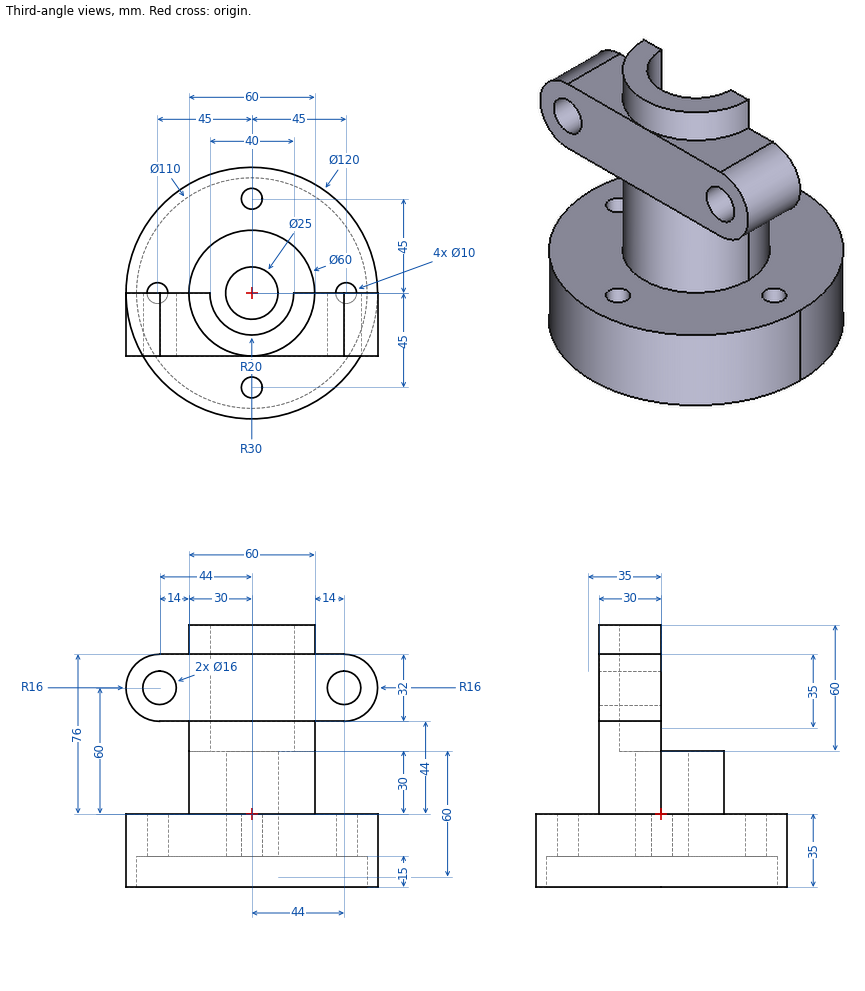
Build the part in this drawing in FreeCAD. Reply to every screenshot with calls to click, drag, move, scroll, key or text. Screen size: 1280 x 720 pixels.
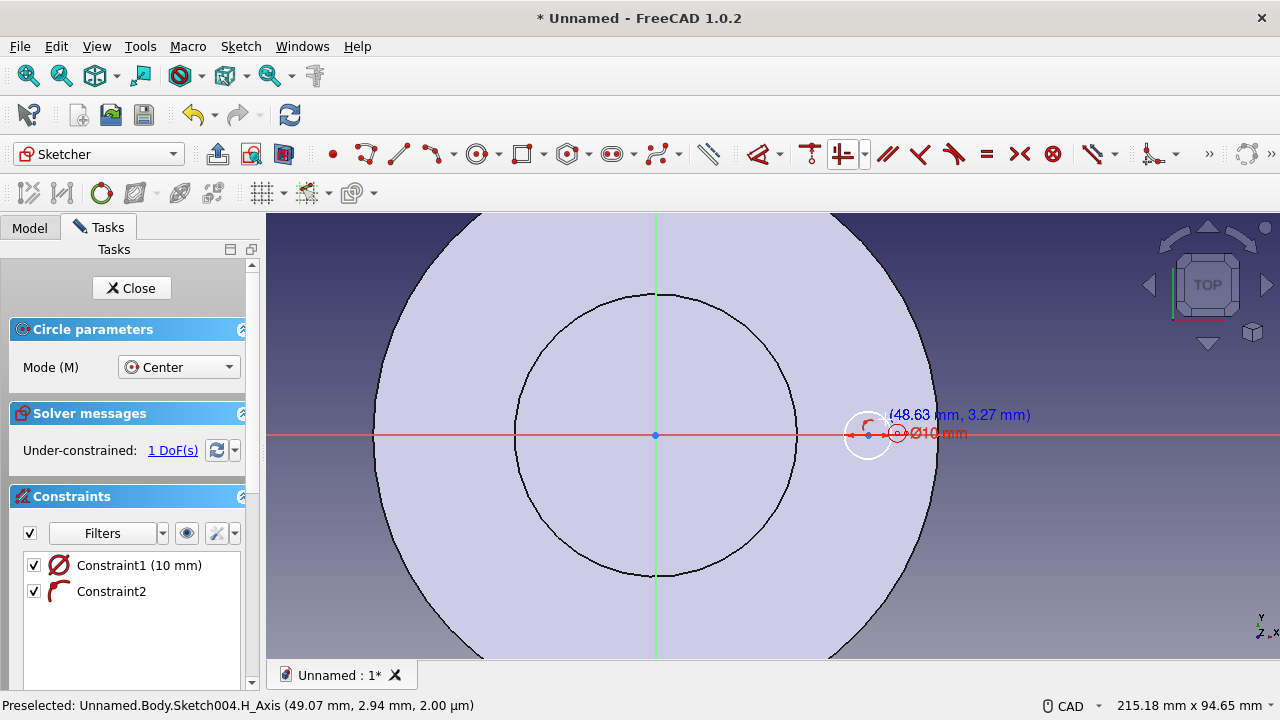
scroll(764, 437, down, 3)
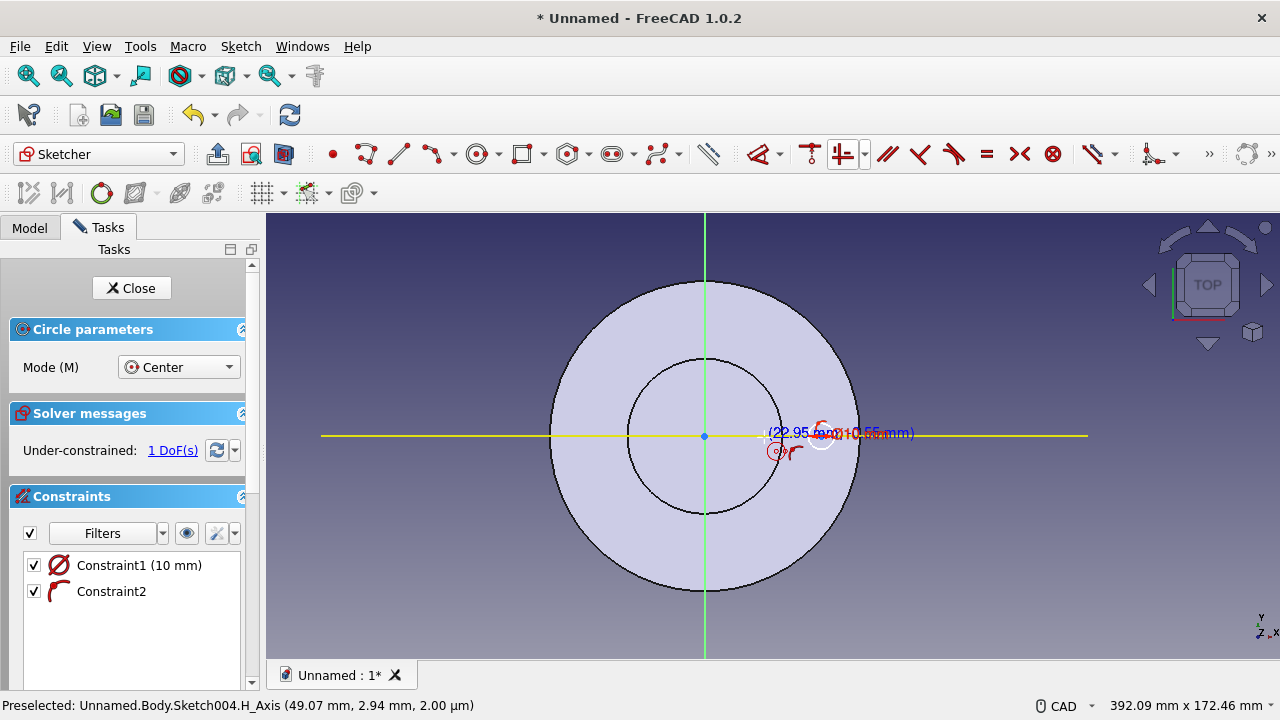
scroll(705, 320, up, 3)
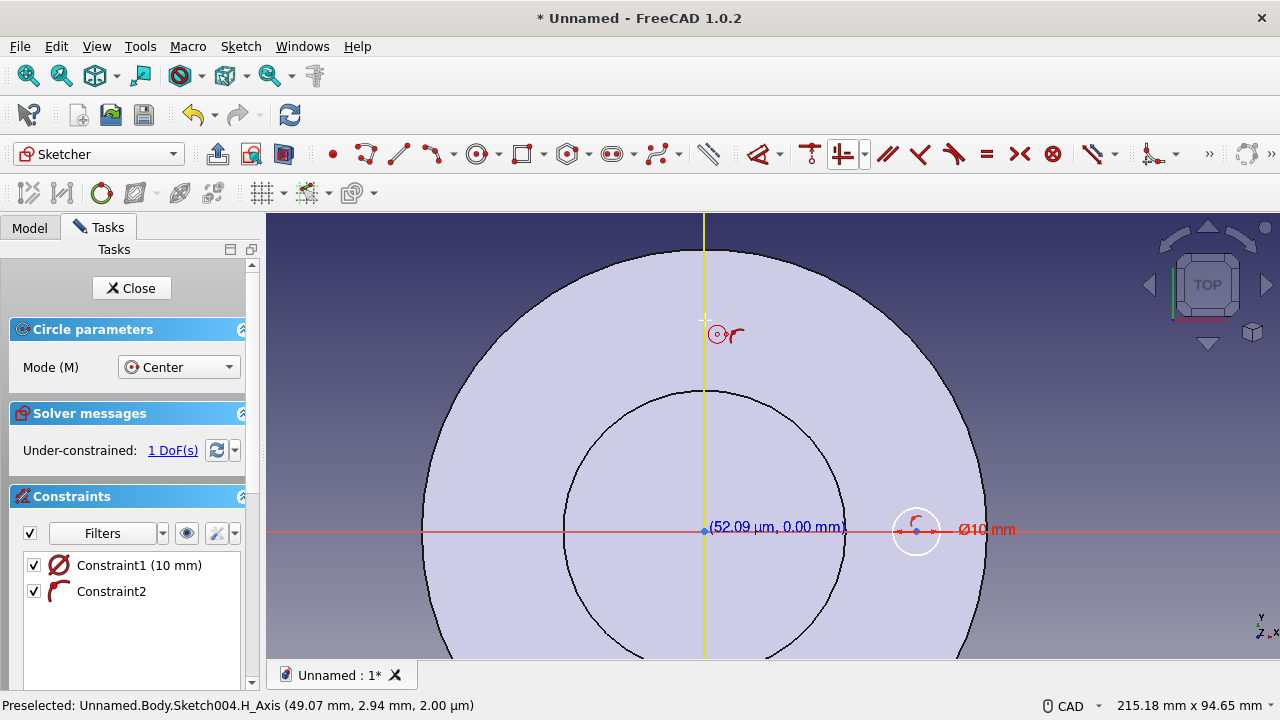
click(704, 320)
move(721, 303)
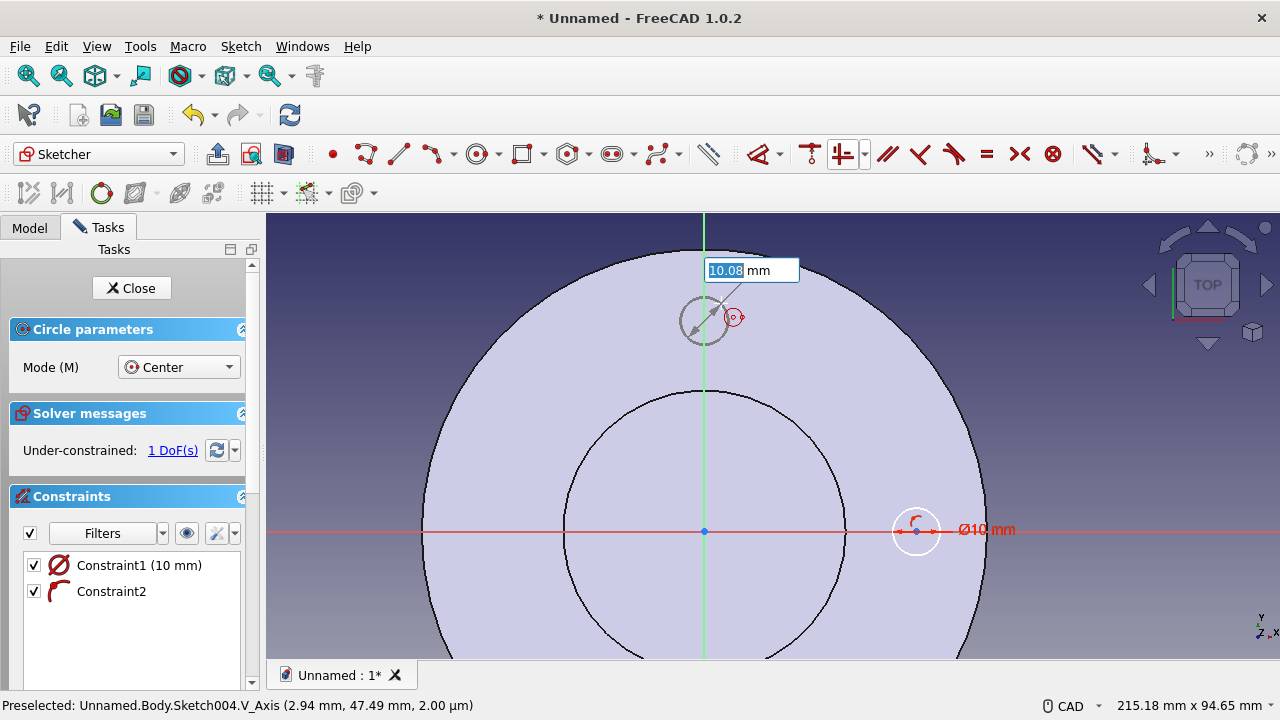
text(10)
key(Return)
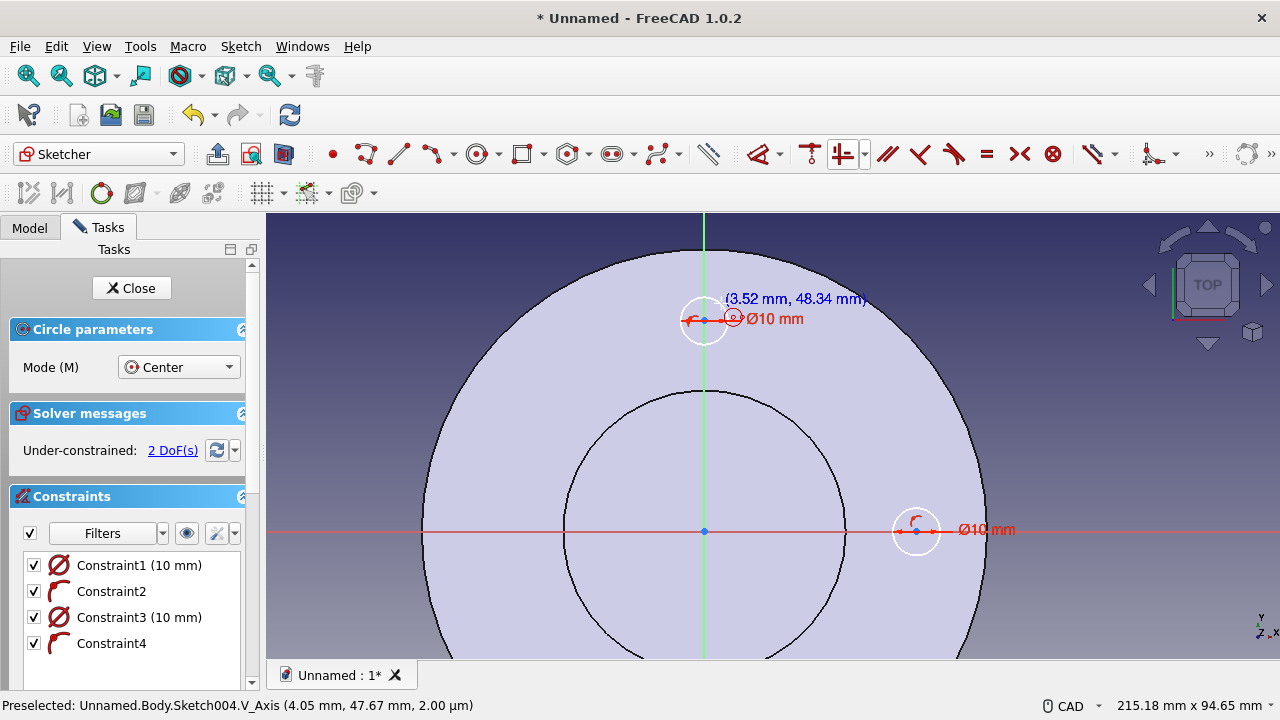
click(492, 532)
move(509, 515)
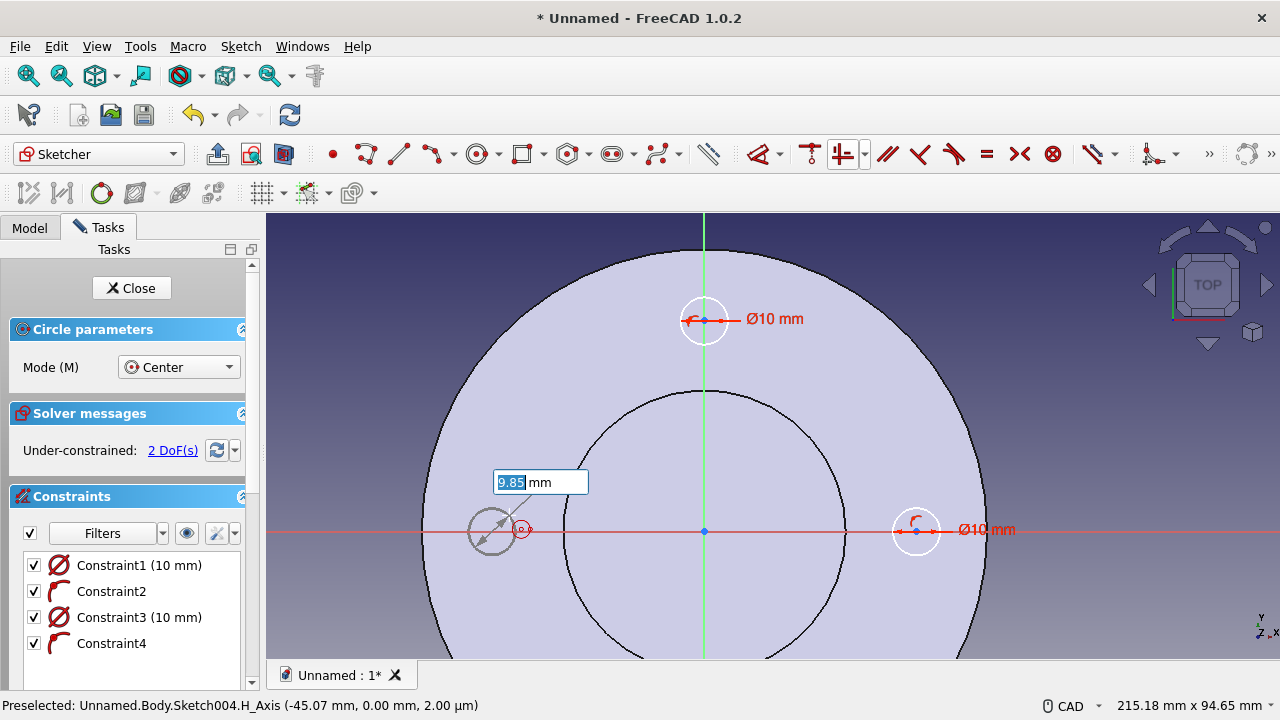
text(10)
key(Return)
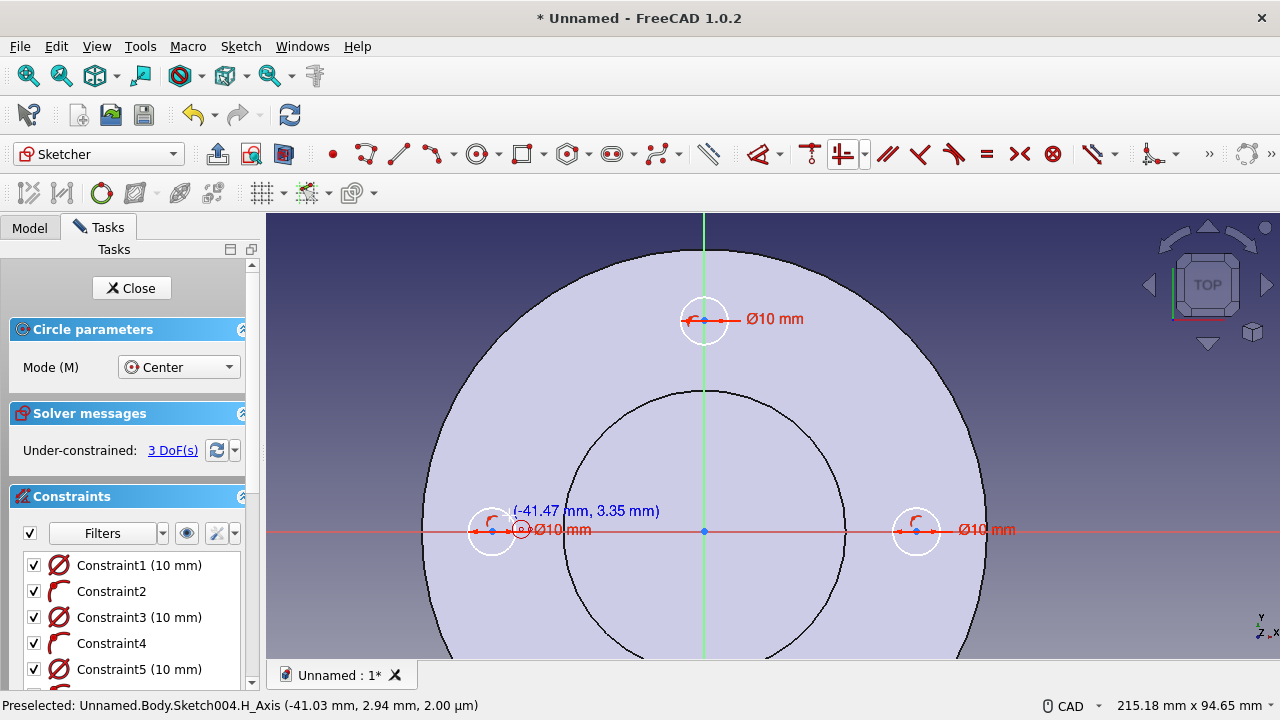
scroll(705, 319, down, 3)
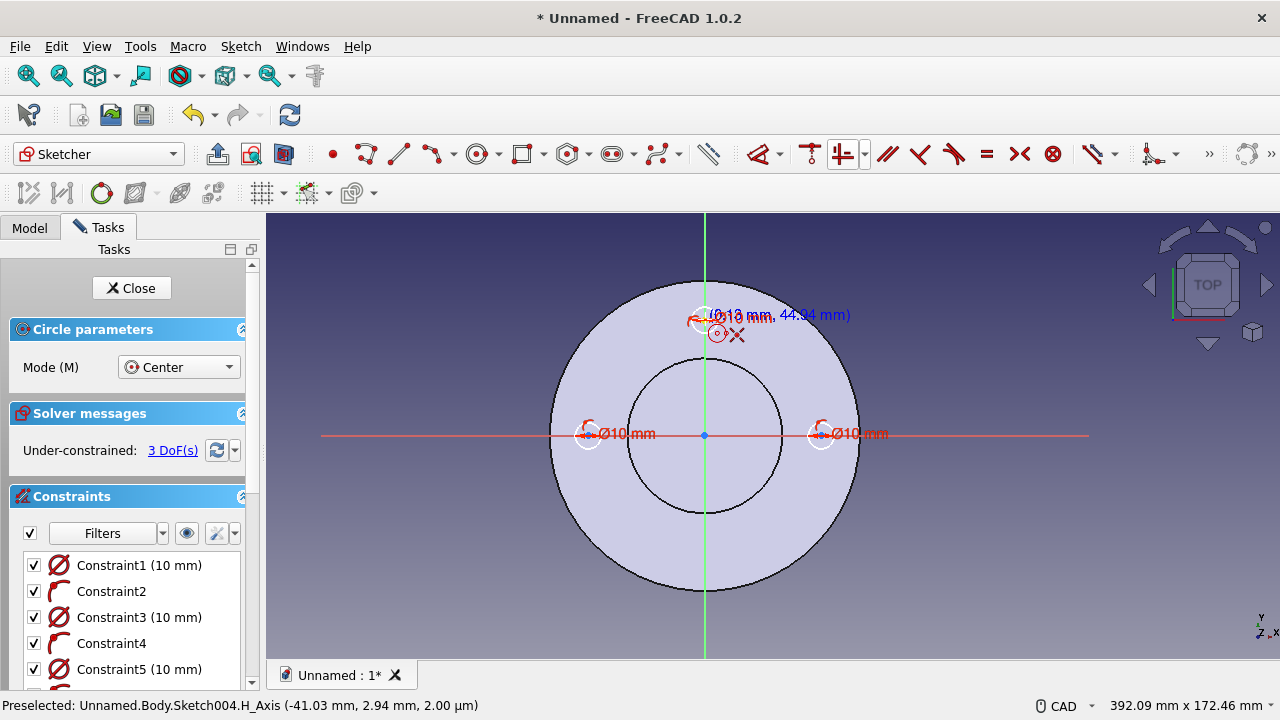
scroll(705, 552, up, 3)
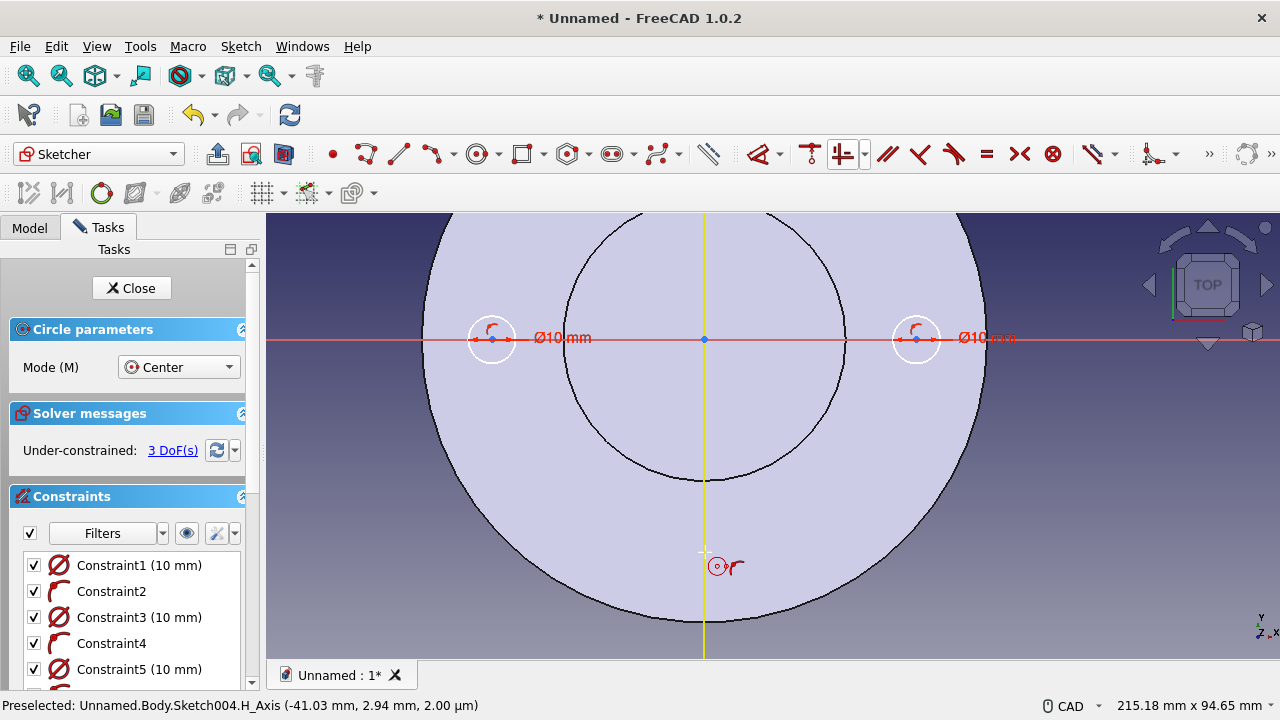
click(704, 552)
move(721, 535)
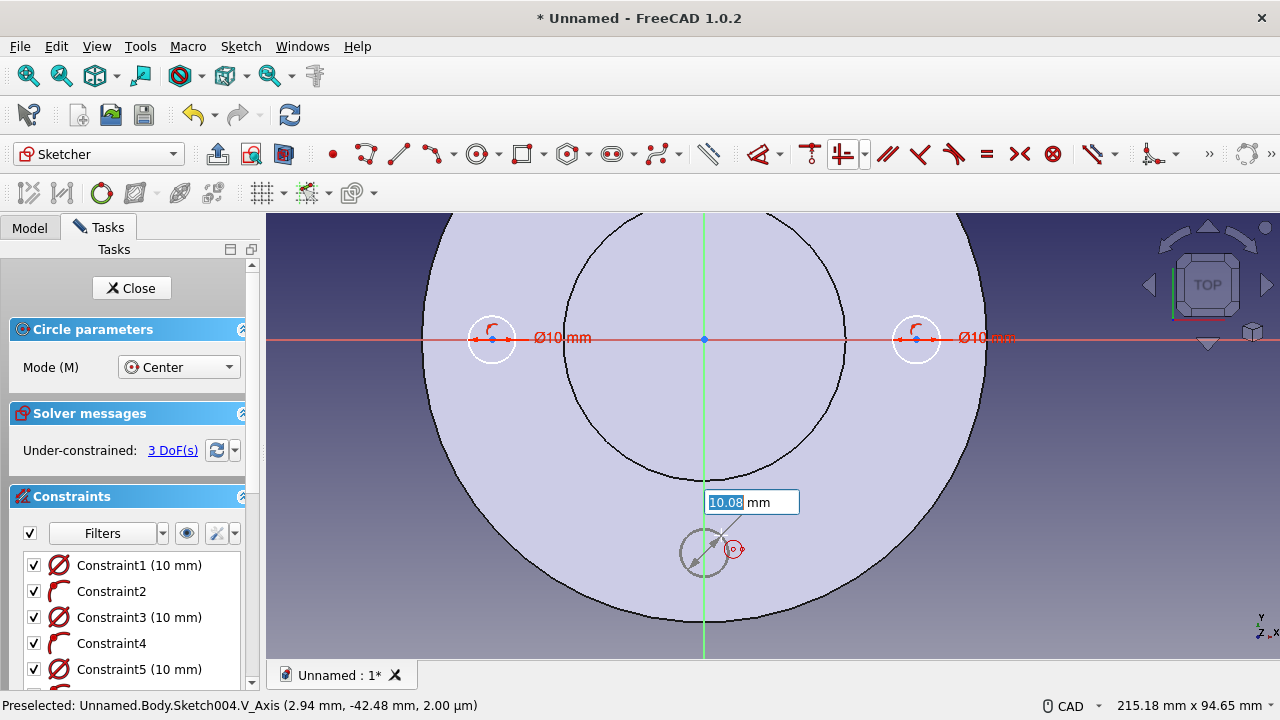
text(10)
key(Return)
key(Escape)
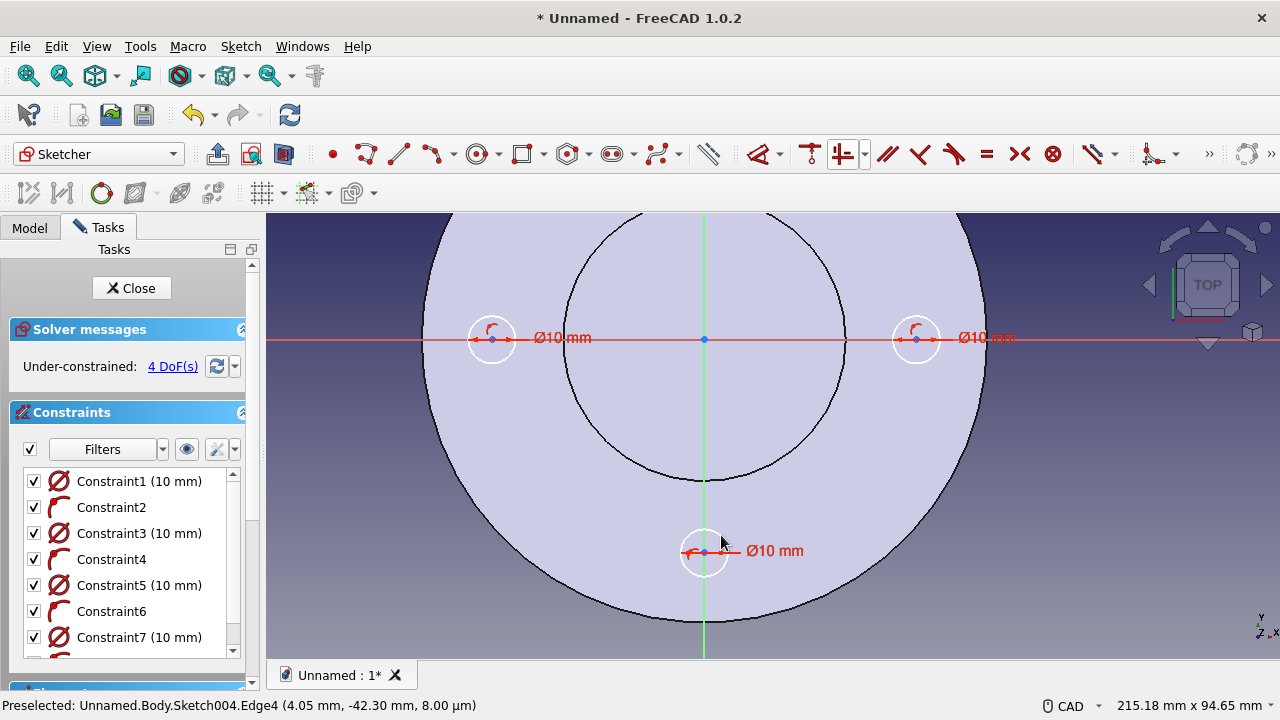
click(758, 154)